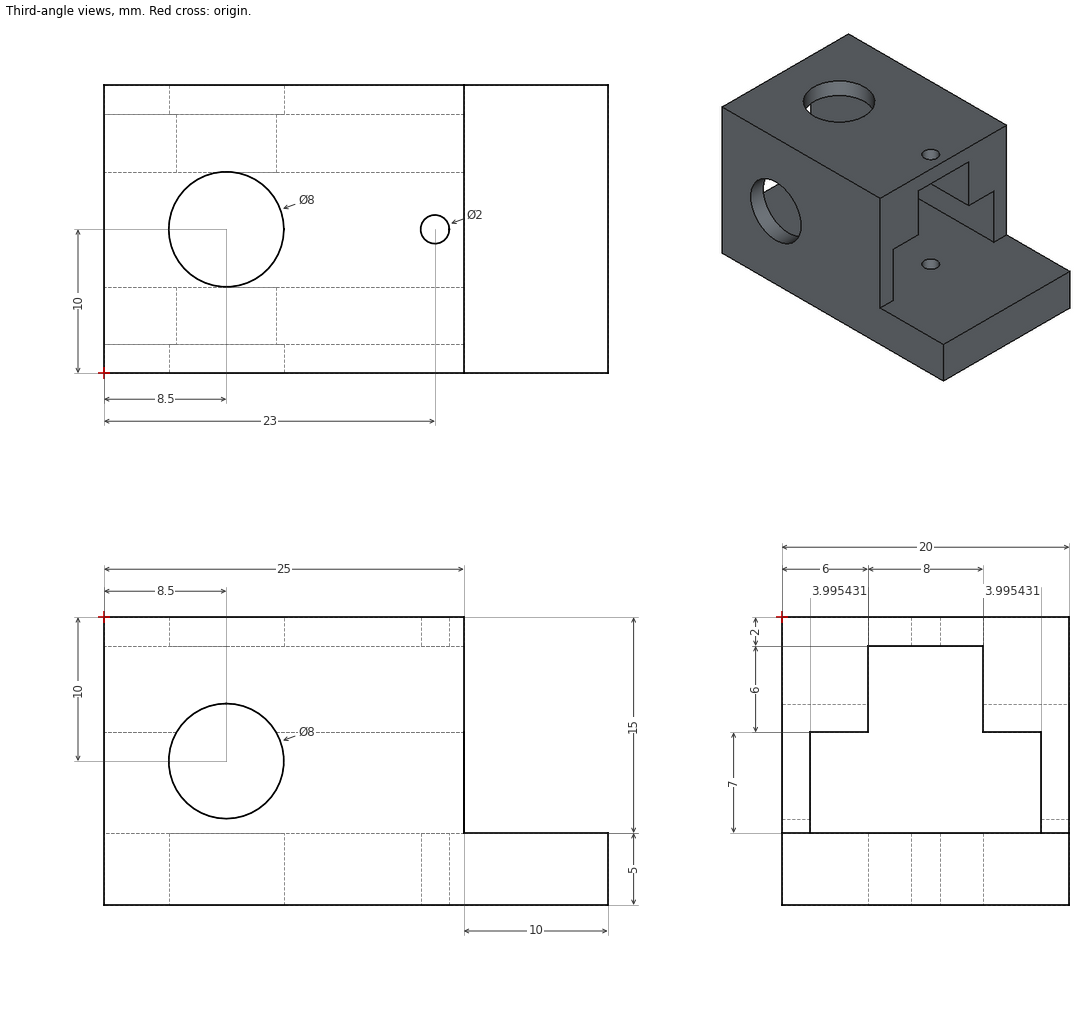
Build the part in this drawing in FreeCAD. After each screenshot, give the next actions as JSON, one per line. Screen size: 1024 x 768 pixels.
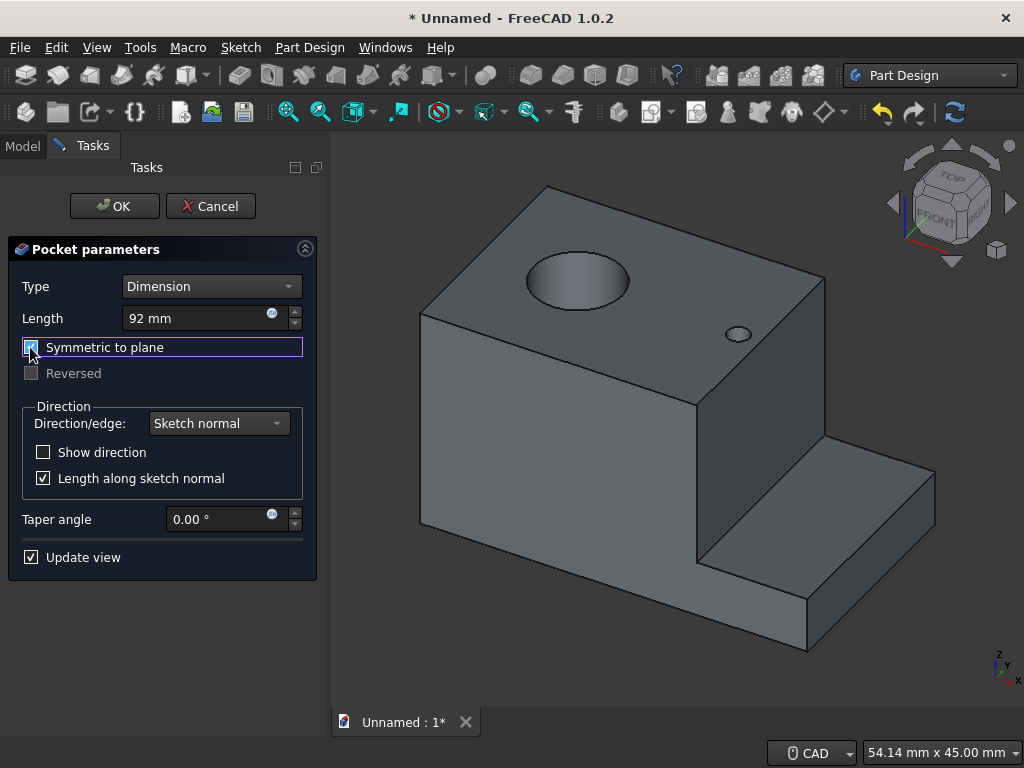
{"action": "left_click", "coordinate": [115, 206]}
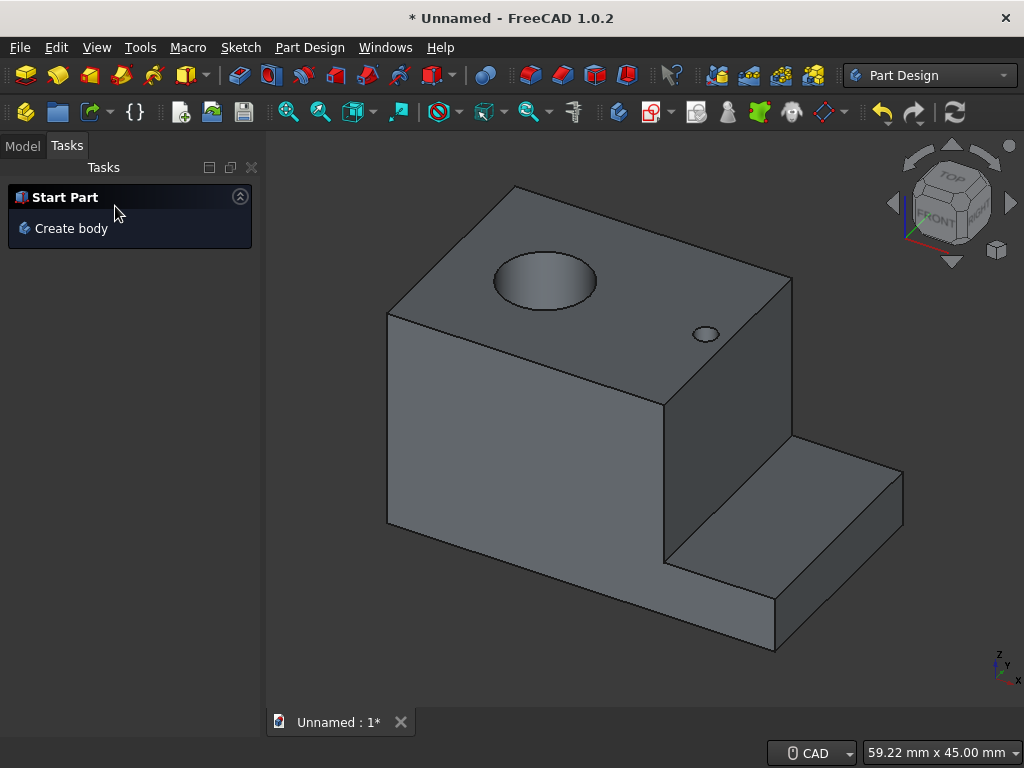
{"action": "key", "text": "4"}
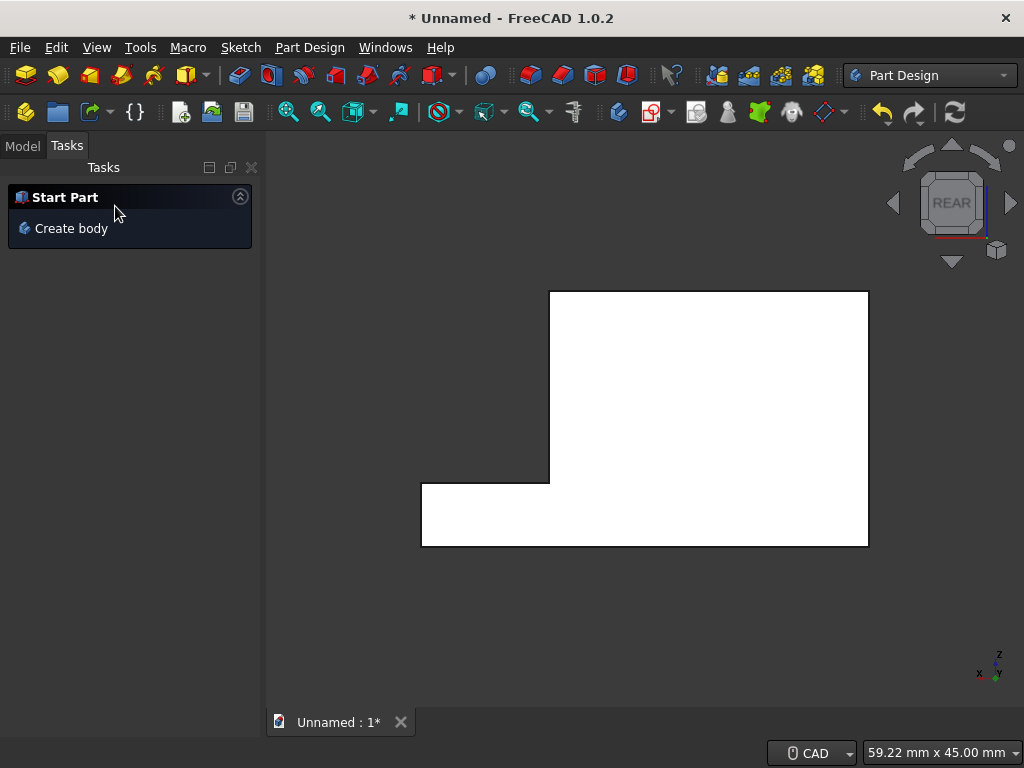
{"action": "left_click", "coordinate": [709, 418]}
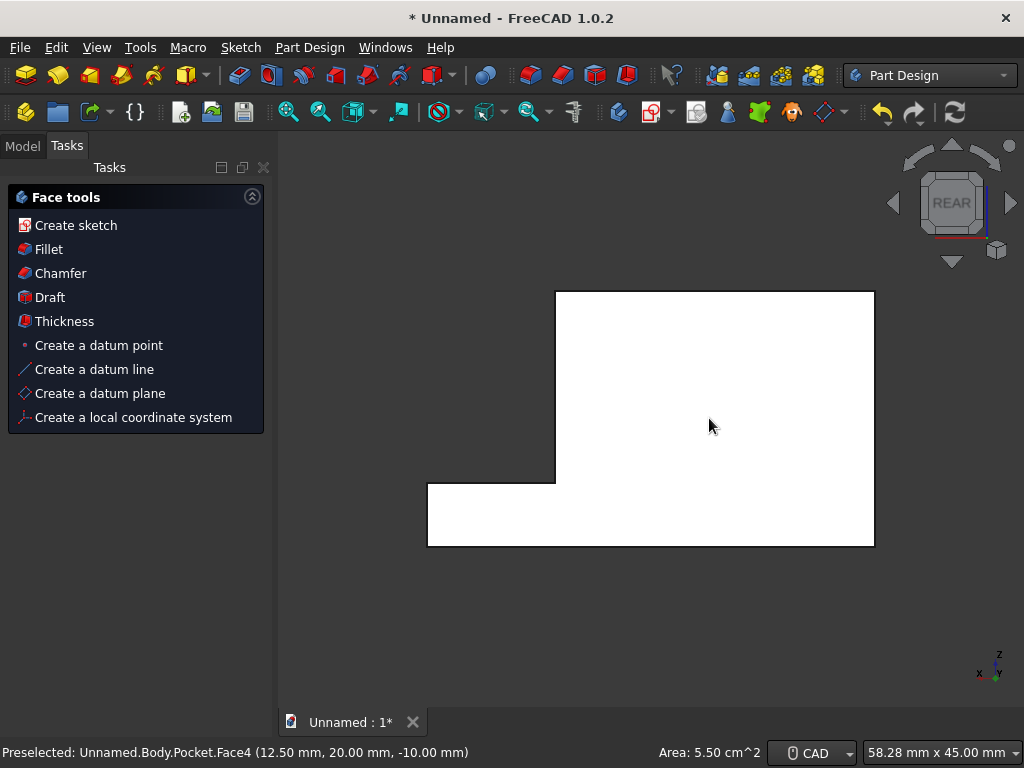
{"action": "left_click", "coordinate": [652, 112]}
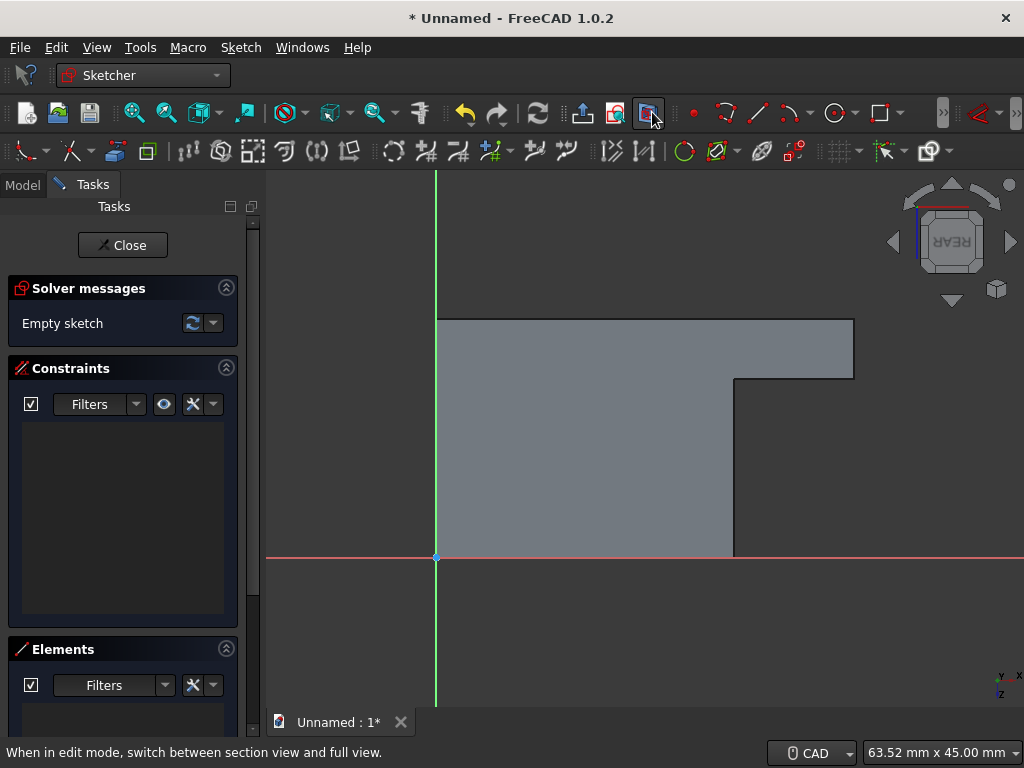
{"action": "scroll", "coordinate": [457, 504], "scroll_direction": "up", "scroll_amount": 4}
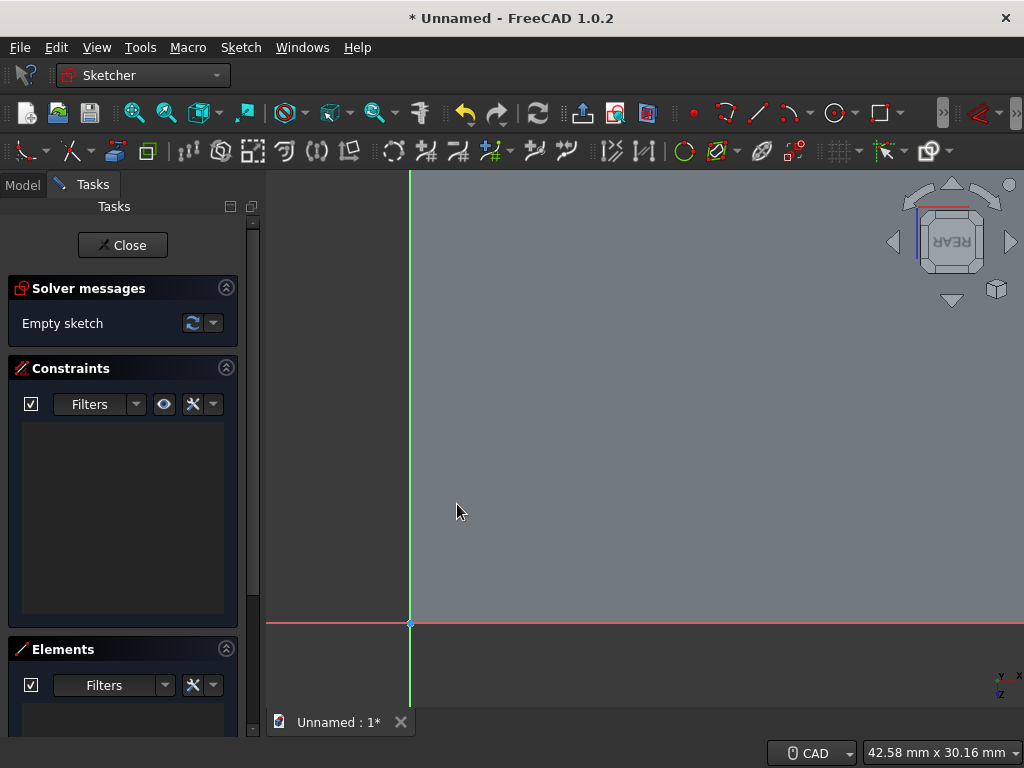
{"action": "key", "text": "g c"}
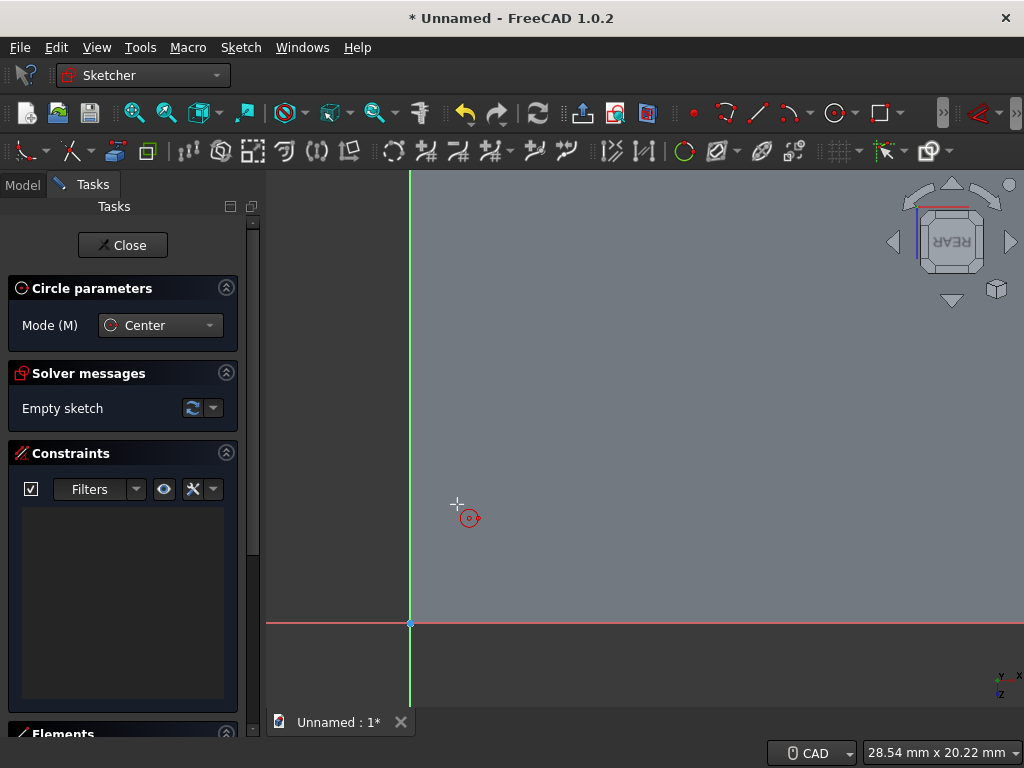
{"action": "left_click", "coordinate": [636, 357]}
{"action": "mouse_move", "coordinate": [711, 282]}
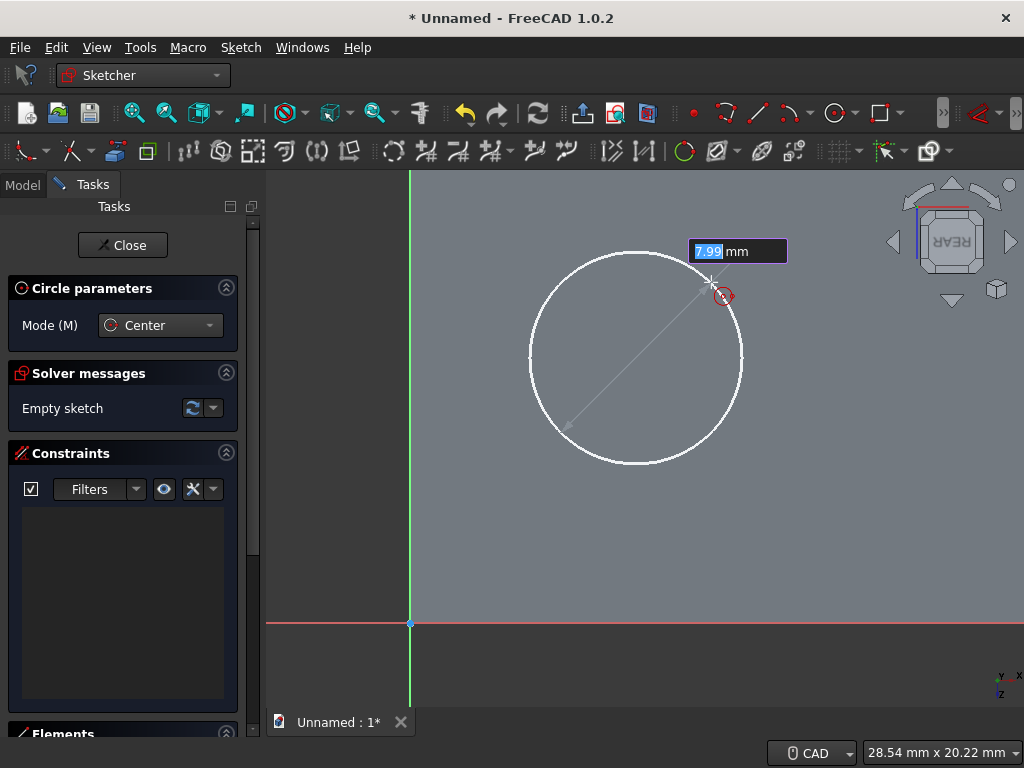
{"action": "type", "text": "8"}
{"action": "key", "text": "Return"}
{"action": "key", "text": "Escape"}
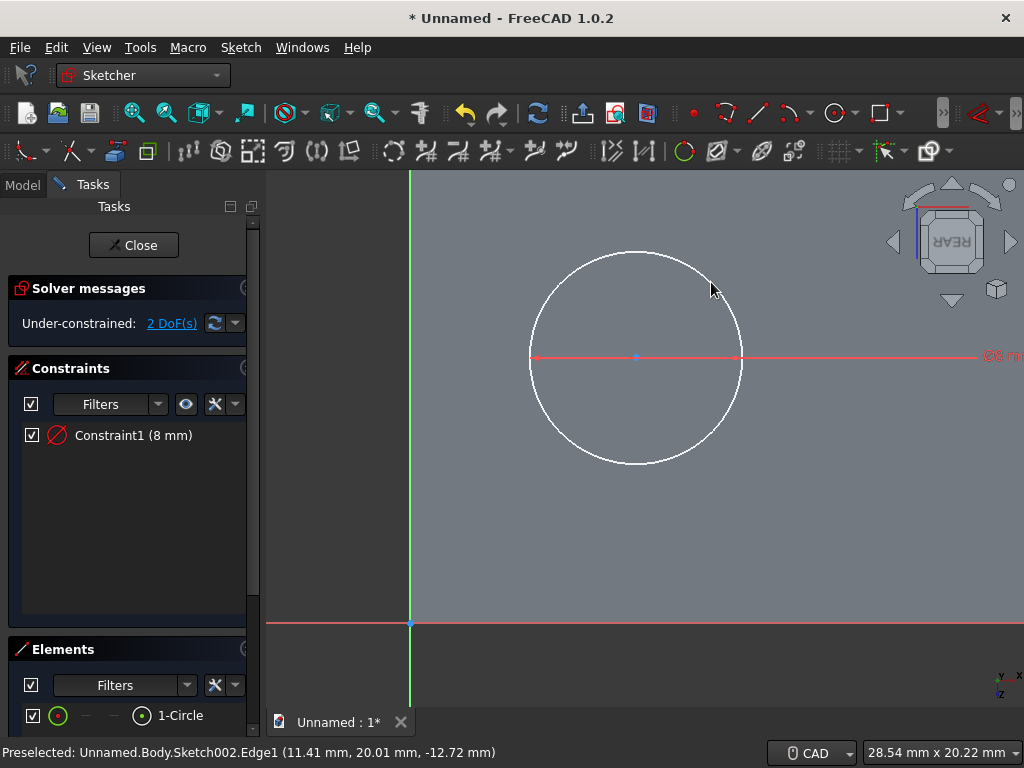
{"action": "left_click", "coordinate": [978, 114]}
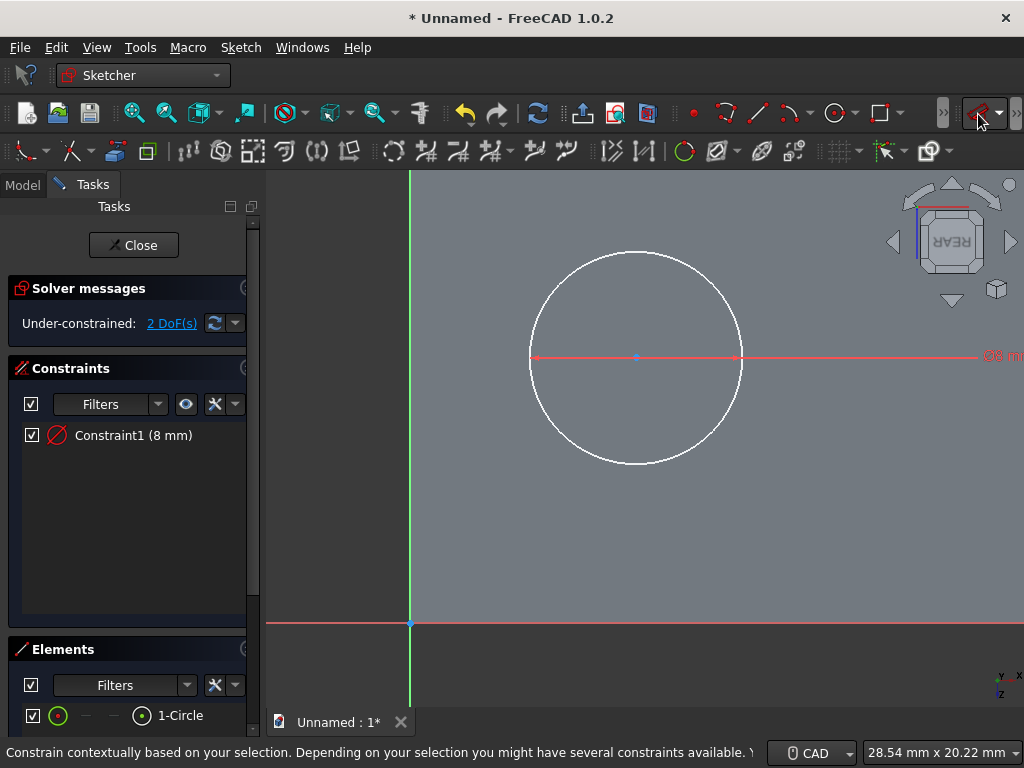
{"action": "left_click", "coordinate": [636, 358]}
{"action": "left_click", "coordinate": [376, 491]}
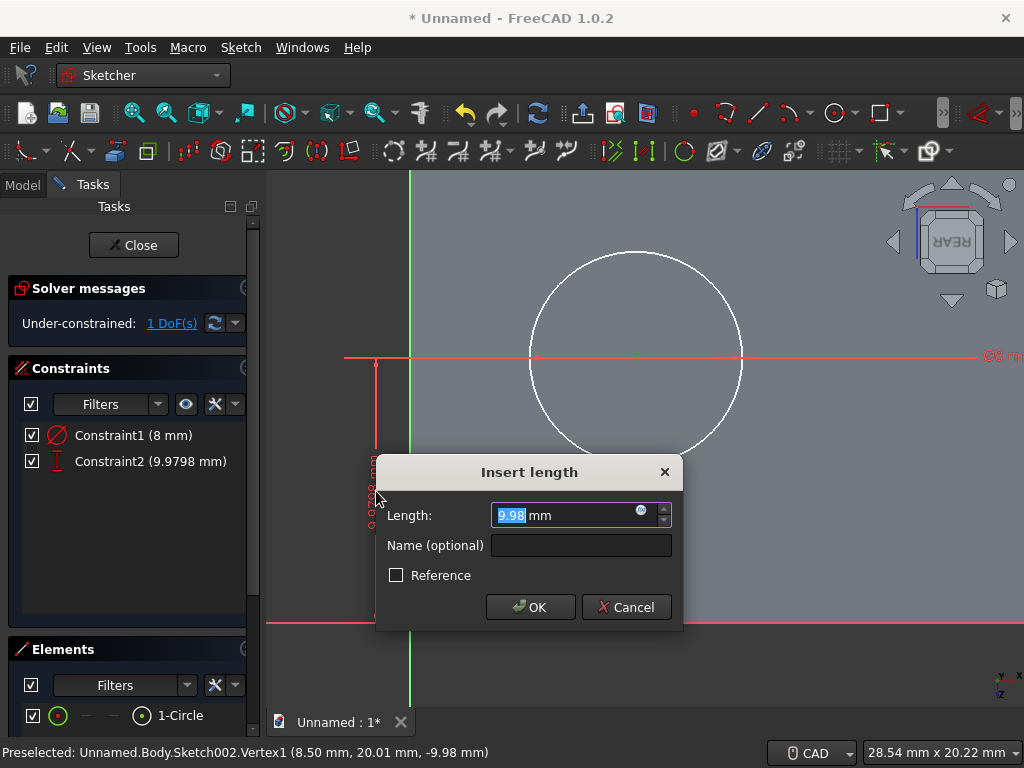
{"action": "type", "text": "10"}
{"action": "key", "text": "Return"}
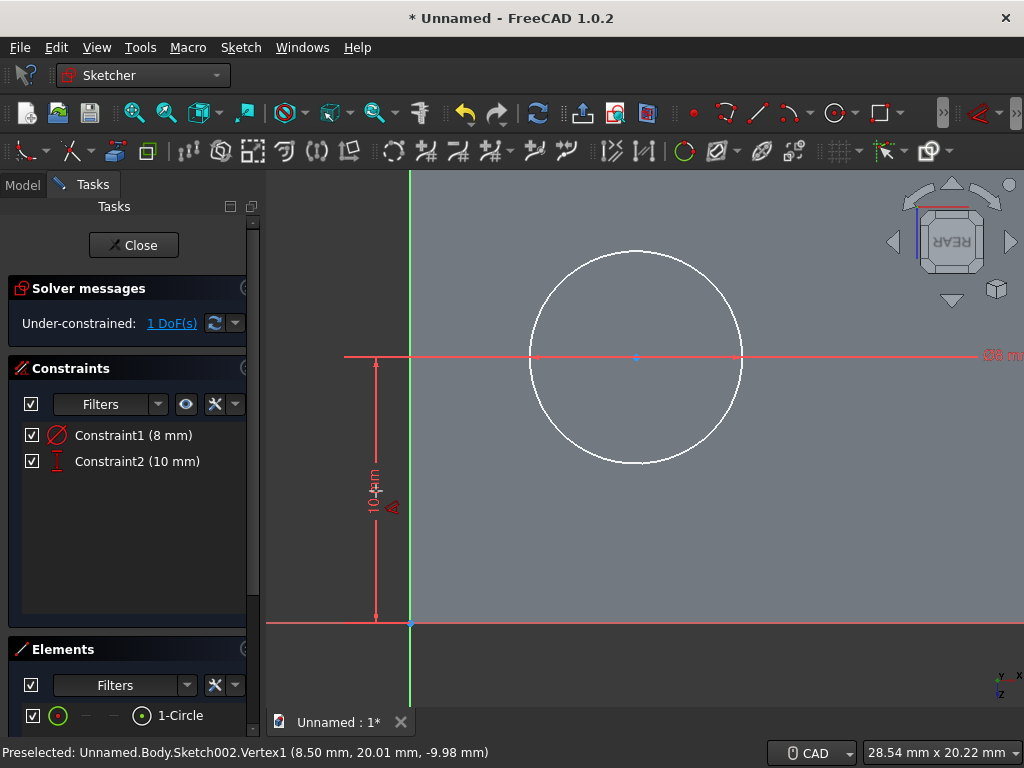
{"action": "left_click", "coordinate": [636, 357]}
{"action": "left_click", "coordinate": [523, 657]}